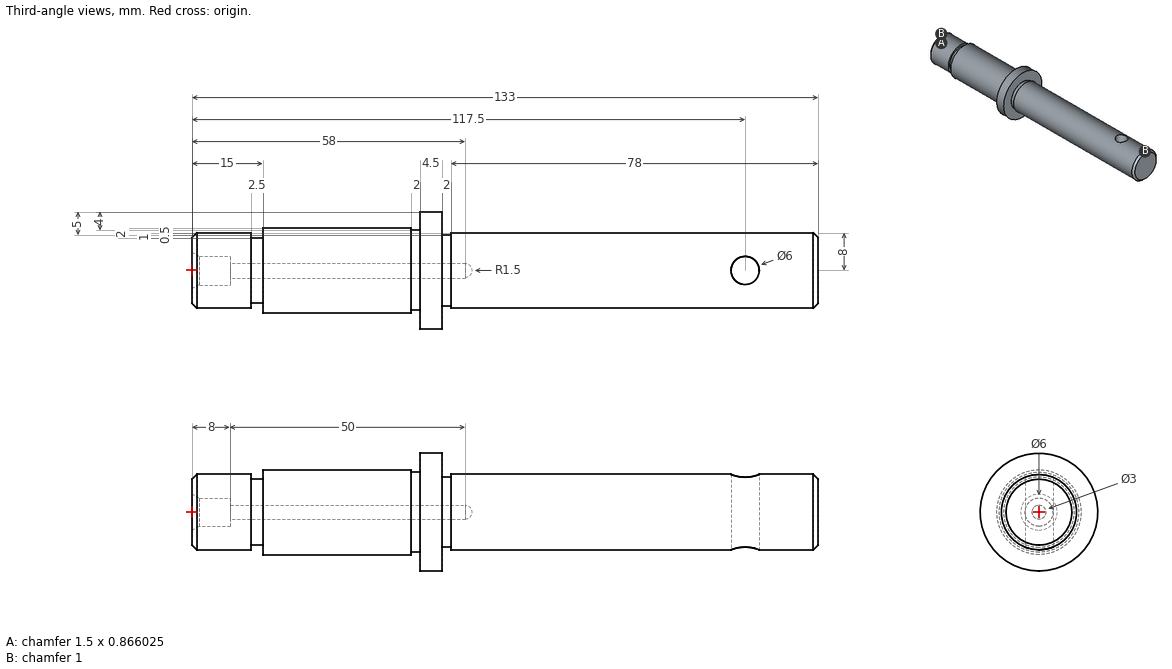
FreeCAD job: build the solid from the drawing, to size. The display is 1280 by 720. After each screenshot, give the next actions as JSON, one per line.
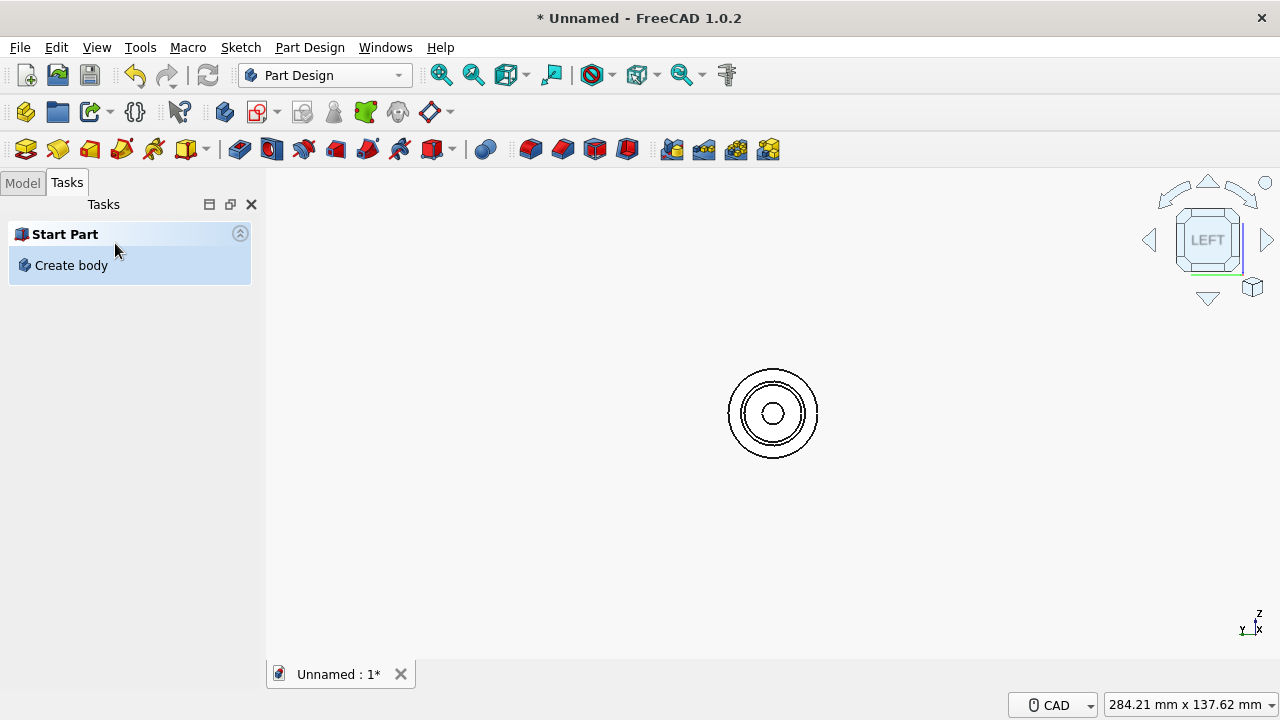
{"action": "left_click", "coordinate": [442, 76]}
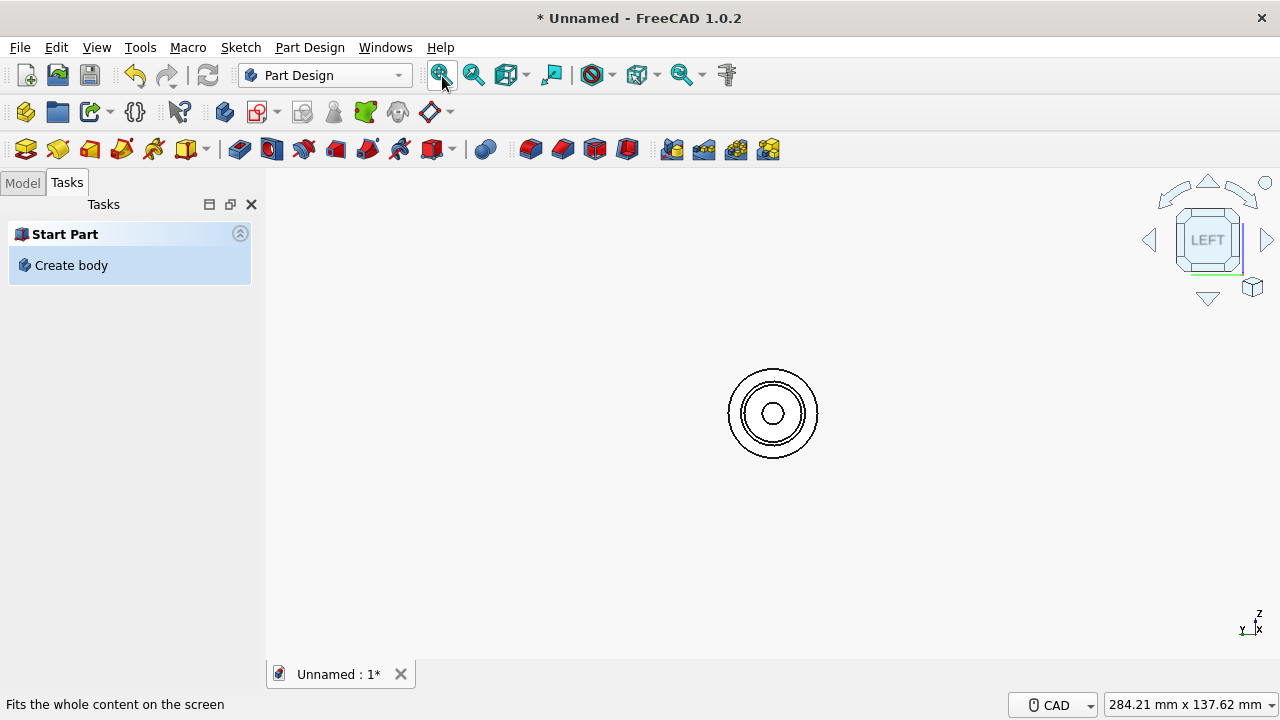
{"action": "left_click", "coordinate": [773, 412]}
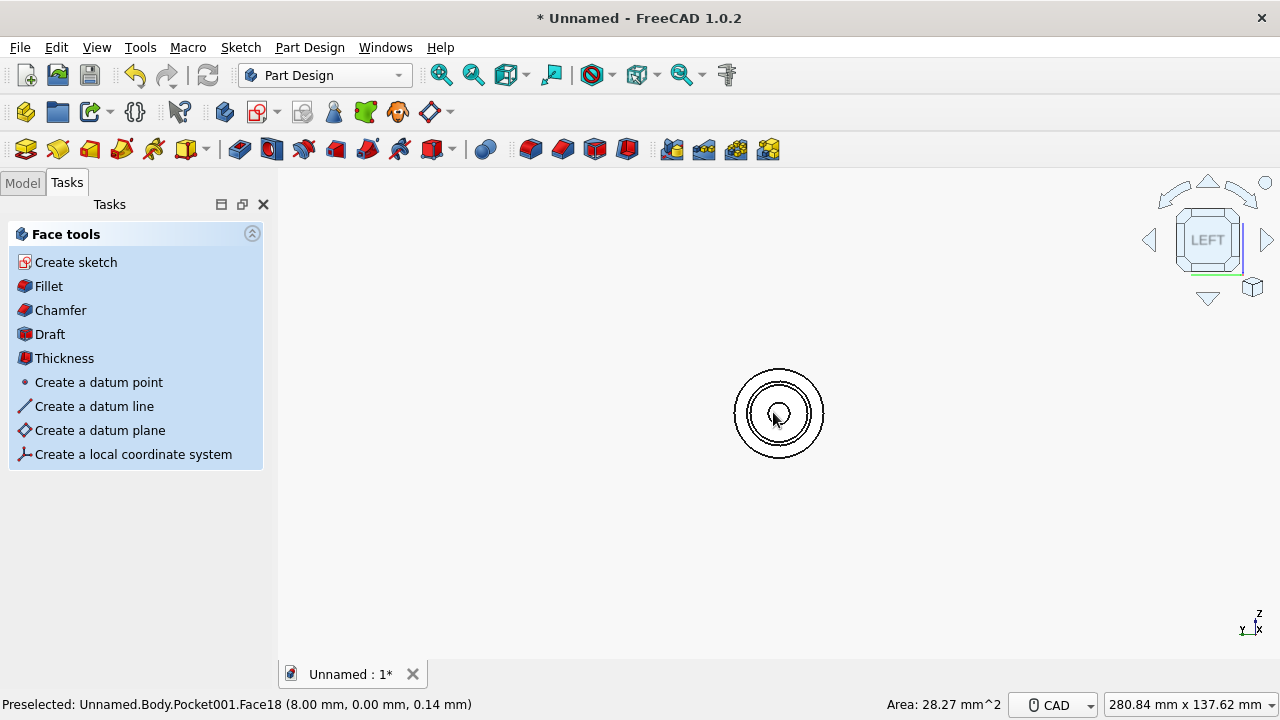
{"action": "left_click", "coordinate": [258, 112]}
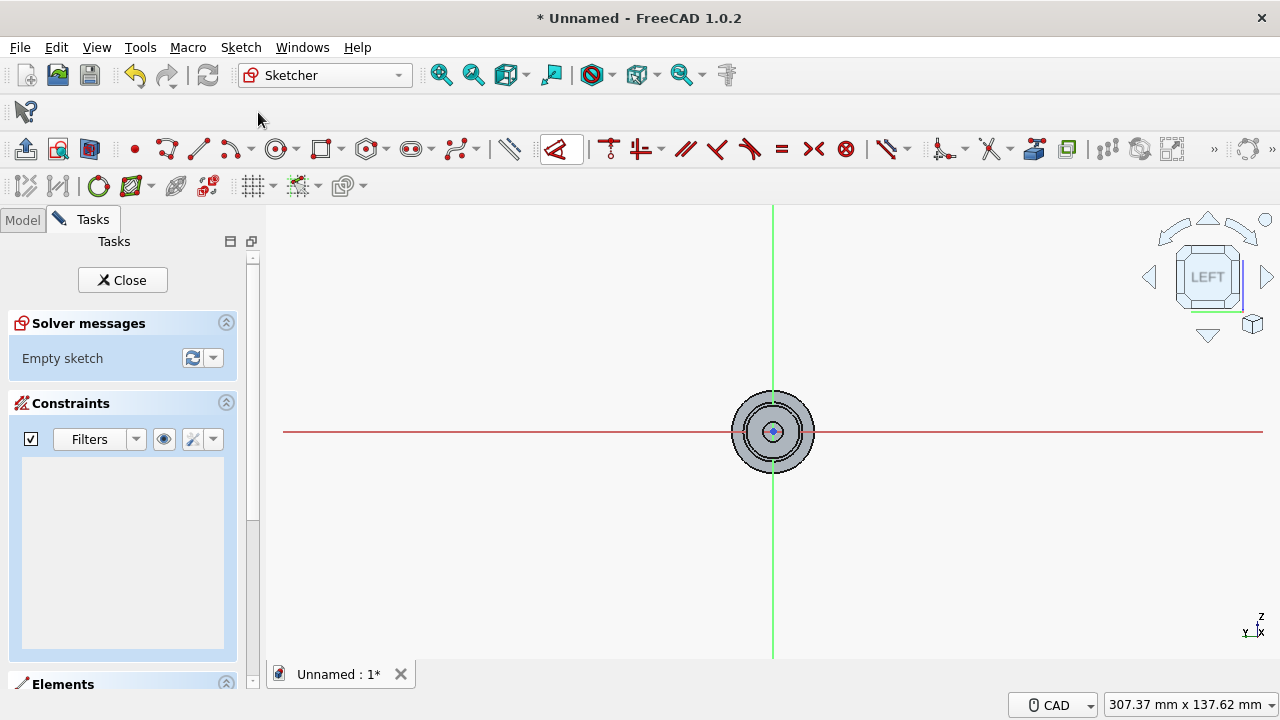
{"action": "left_click", "coordinate": [90, 150]}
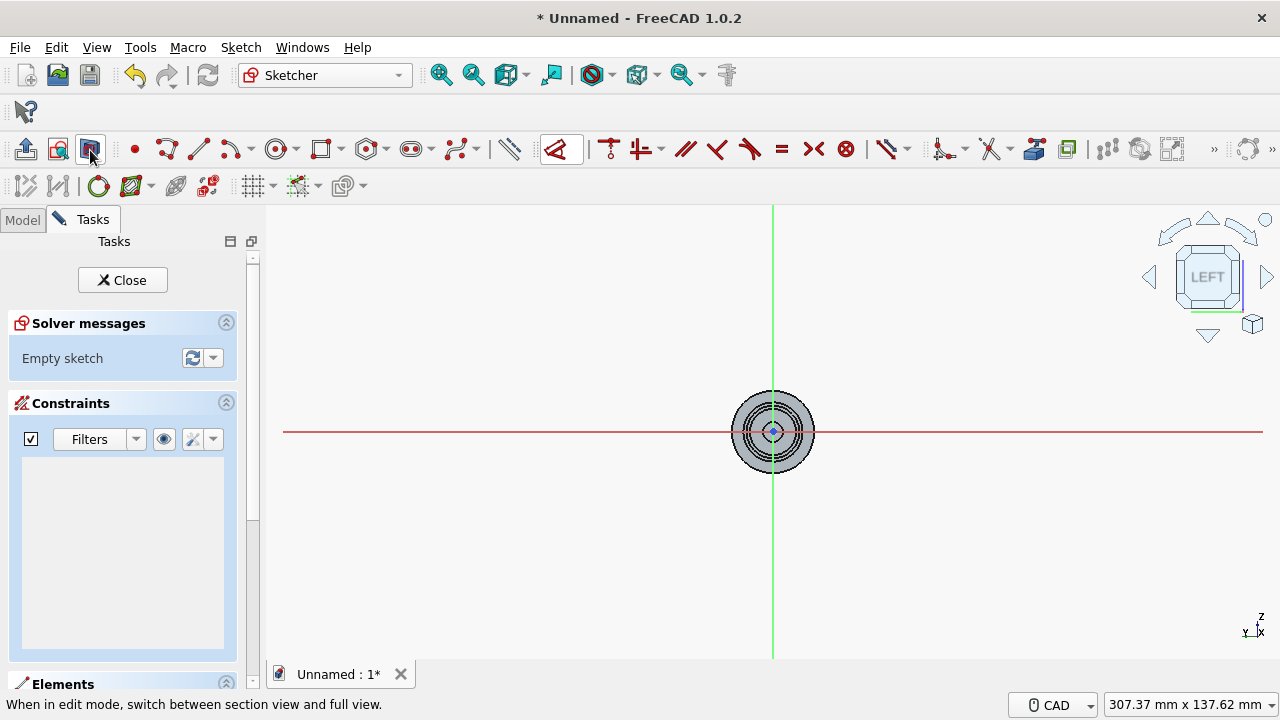
{"action": "scroll", "coordinate": [777, 432], "scroll_direction": "up", "scroll_amount": 15}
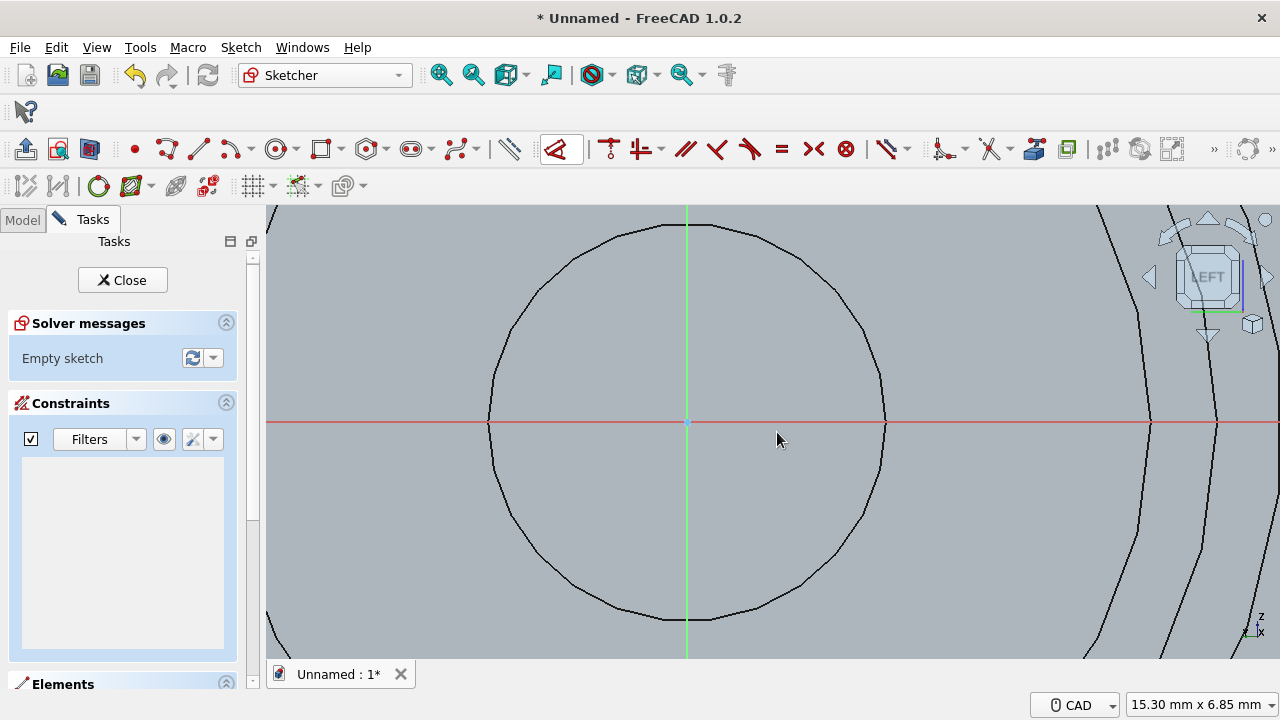
{"action": "scroll", "coordinate": [652, 403], "scroll_direction": "up", "scroll_amount": 2}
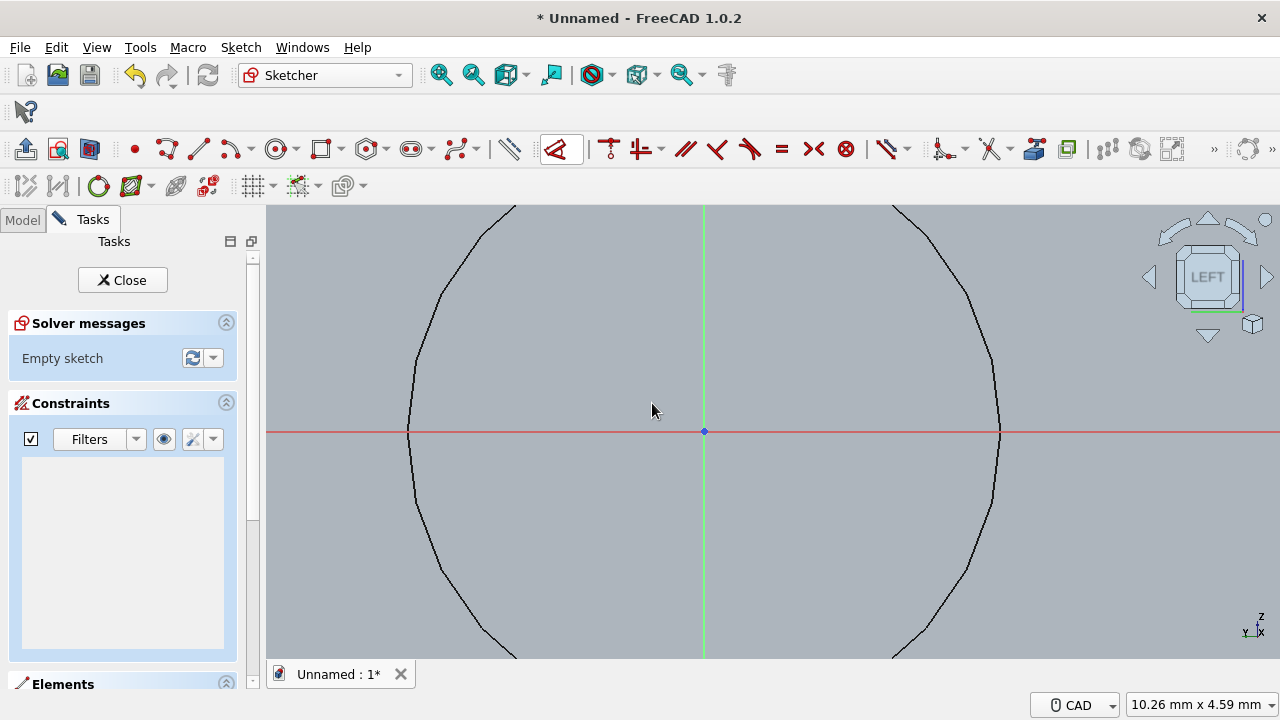
{"action": "left_click", "coordinate": [276, 150]}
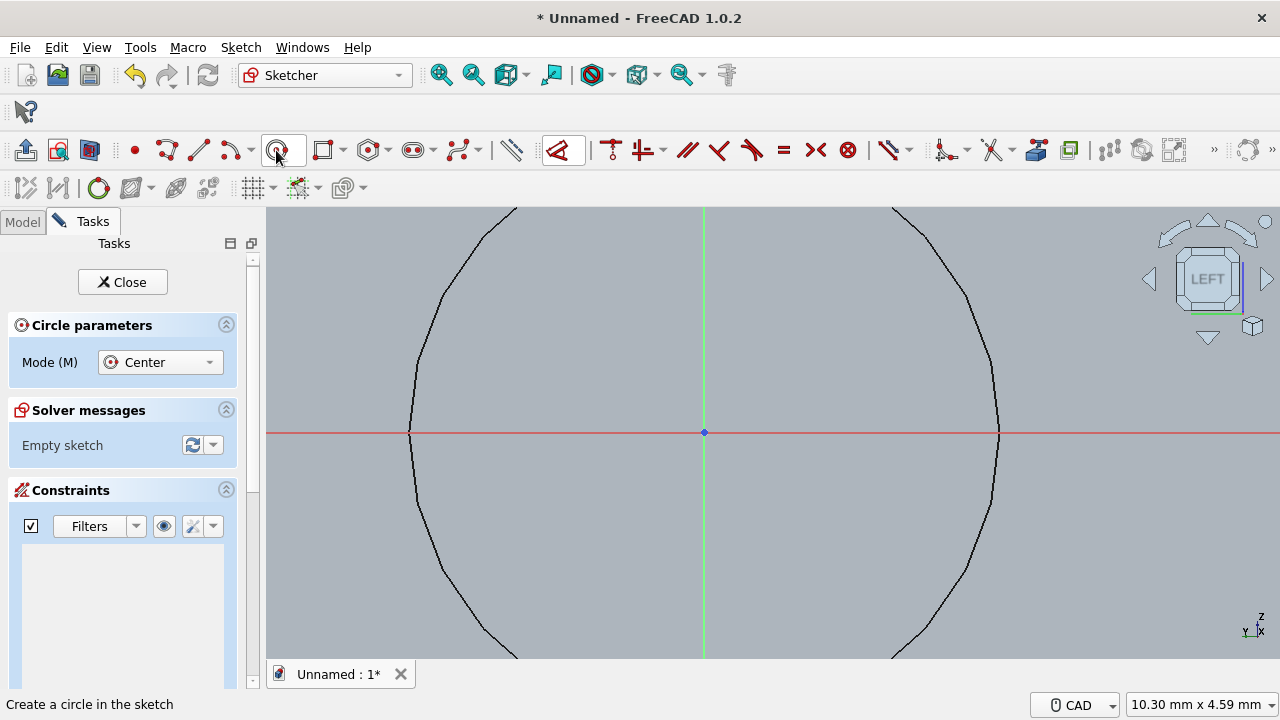
{"action": "left_click", "coordinate": [704, 433]}
{"action": "mouse_move", "coordinate": [809, 328]}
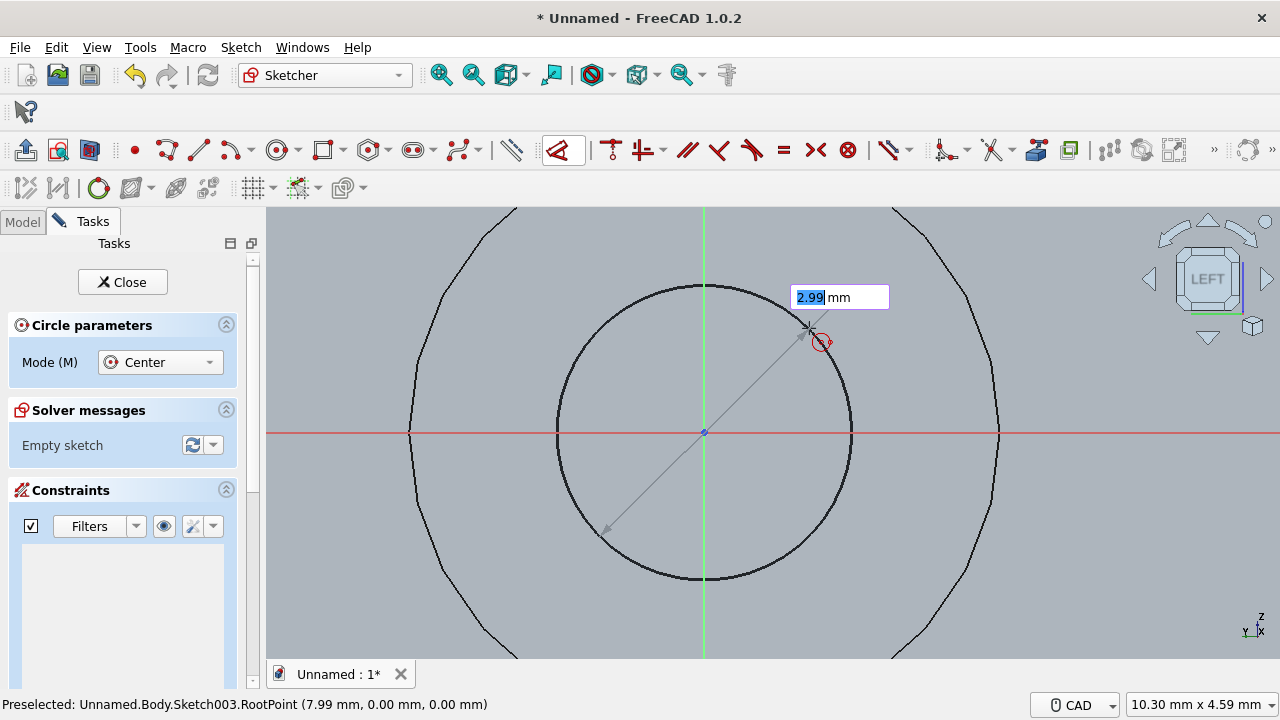
{"action": "type", "text": "3"}
{"action": "key", "text": "Return"}
{"action": "key", "text": "Escape"}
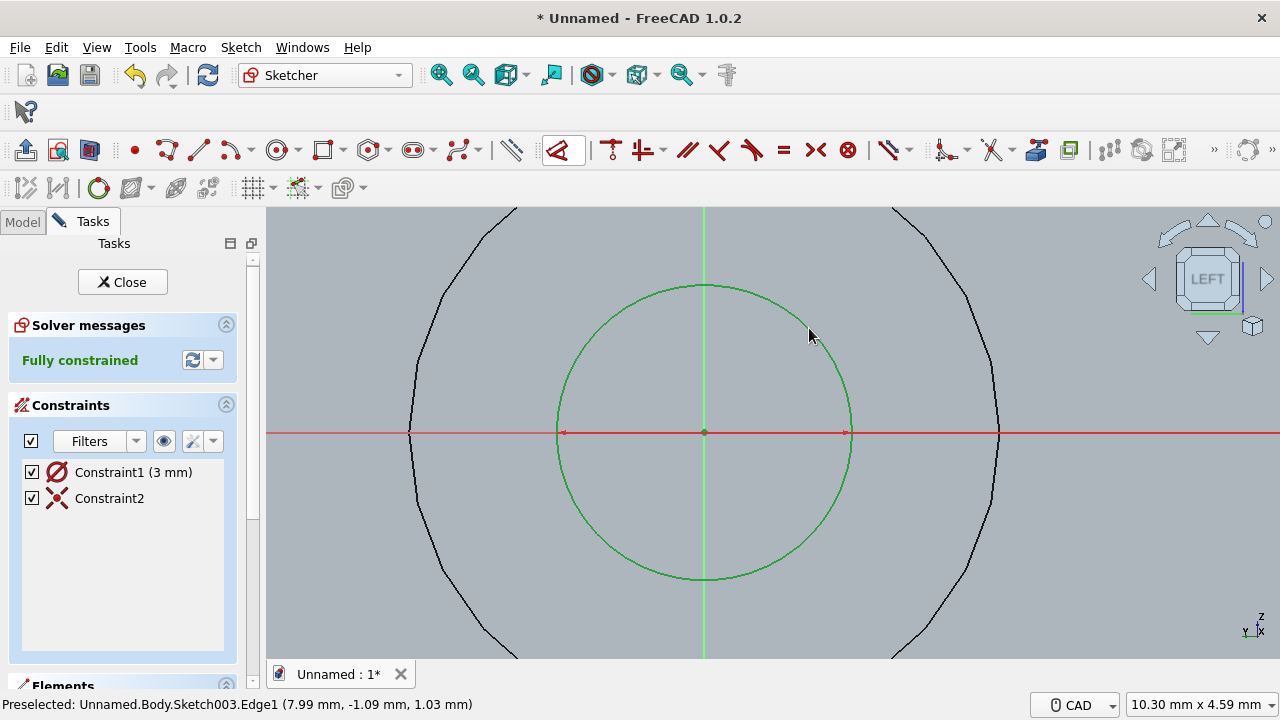
{"action": "left_click", "coordinate": [123, 282]}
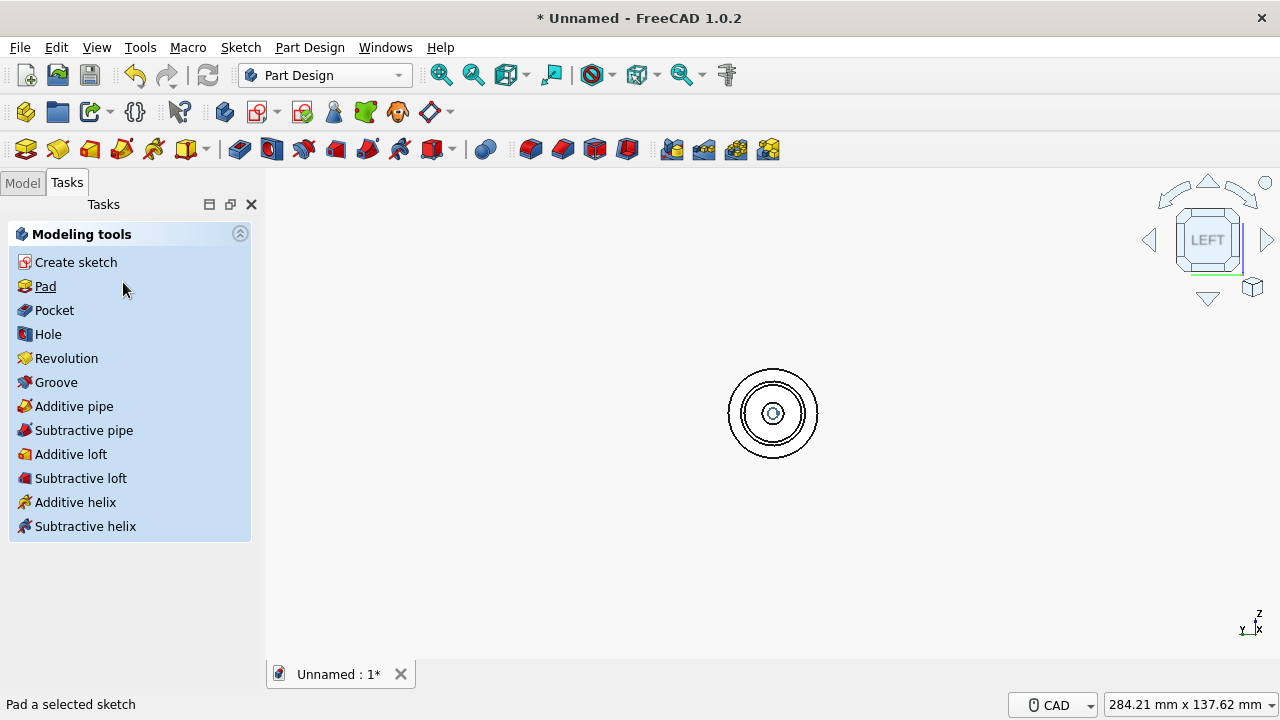
{"action": "left_click", "coordinate": [240, 150]}